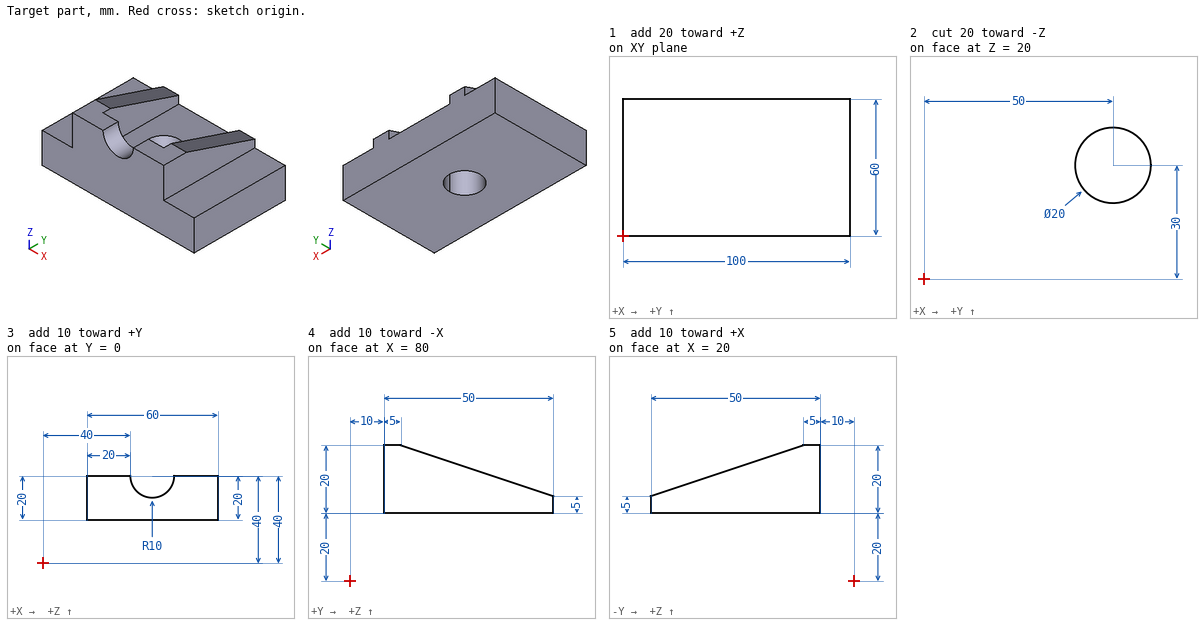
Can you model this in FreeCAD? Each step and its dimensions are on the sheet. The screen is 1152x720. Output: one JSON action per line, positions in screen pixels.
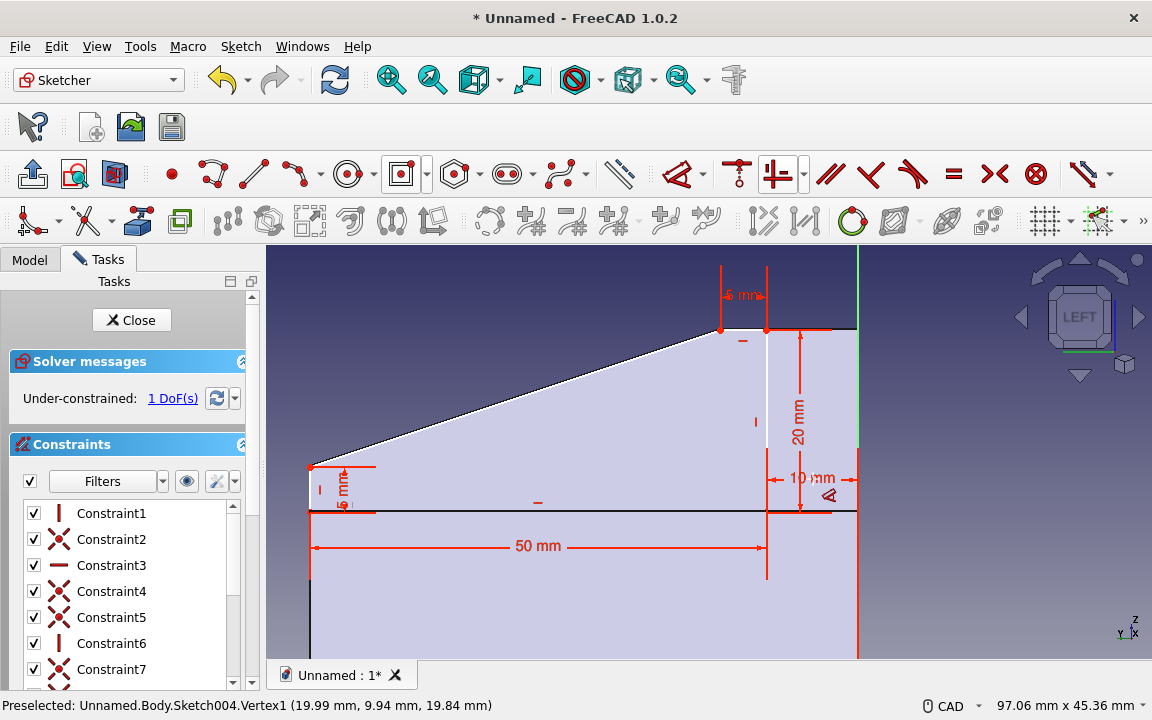
{"action": "left_click", "coordinate": [767, 513]}
{"action": "left_click", "coordinate": [892, 572]}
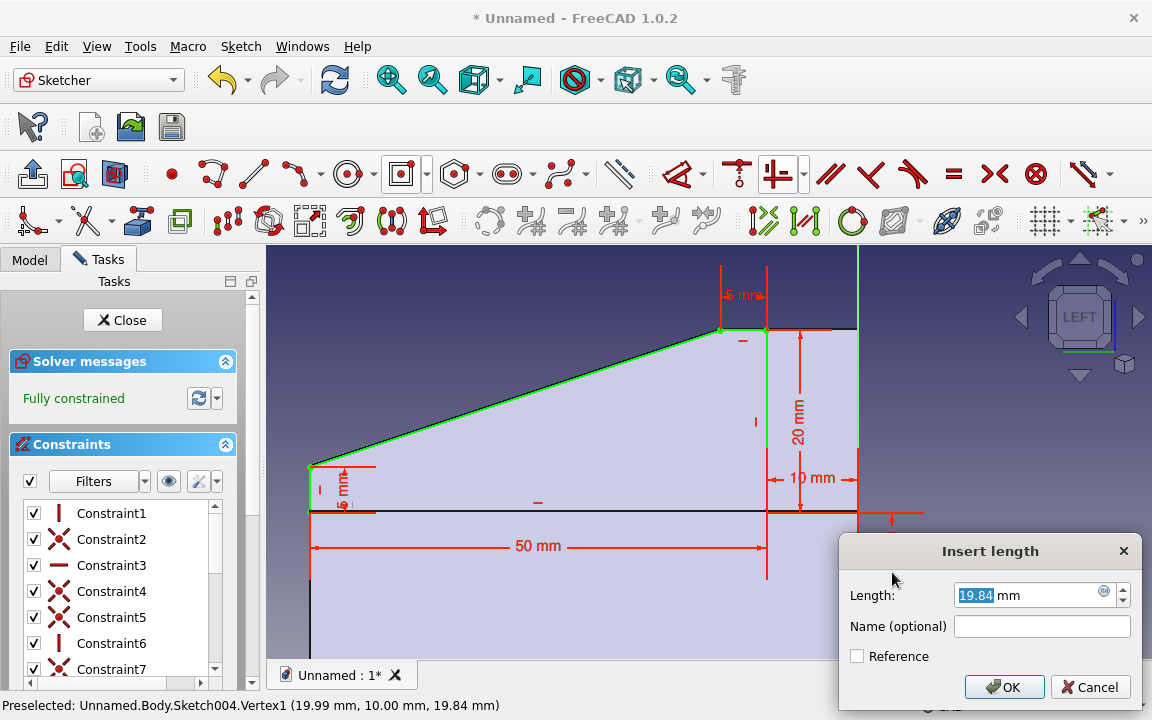
{"action": "type", "text": "20"}
{"action": "key", "text": "Return"}
{"action": "key", "text": "Escape"}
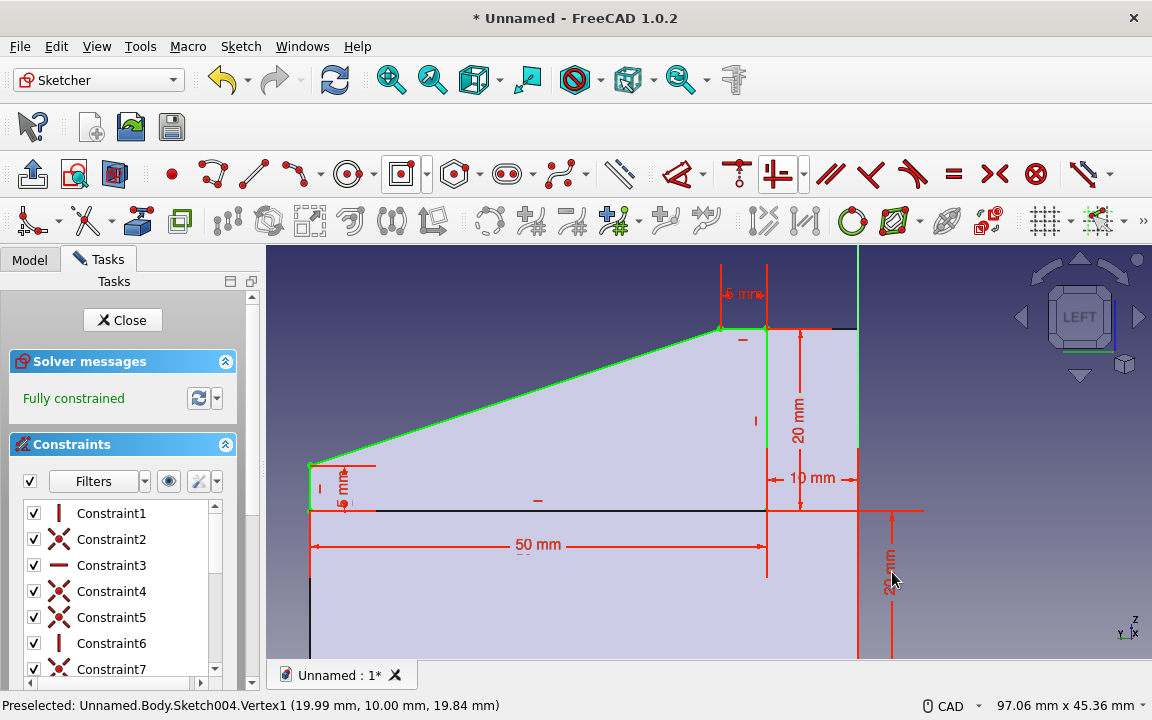
{"action": "left_click", "coordinate": [123, 320]}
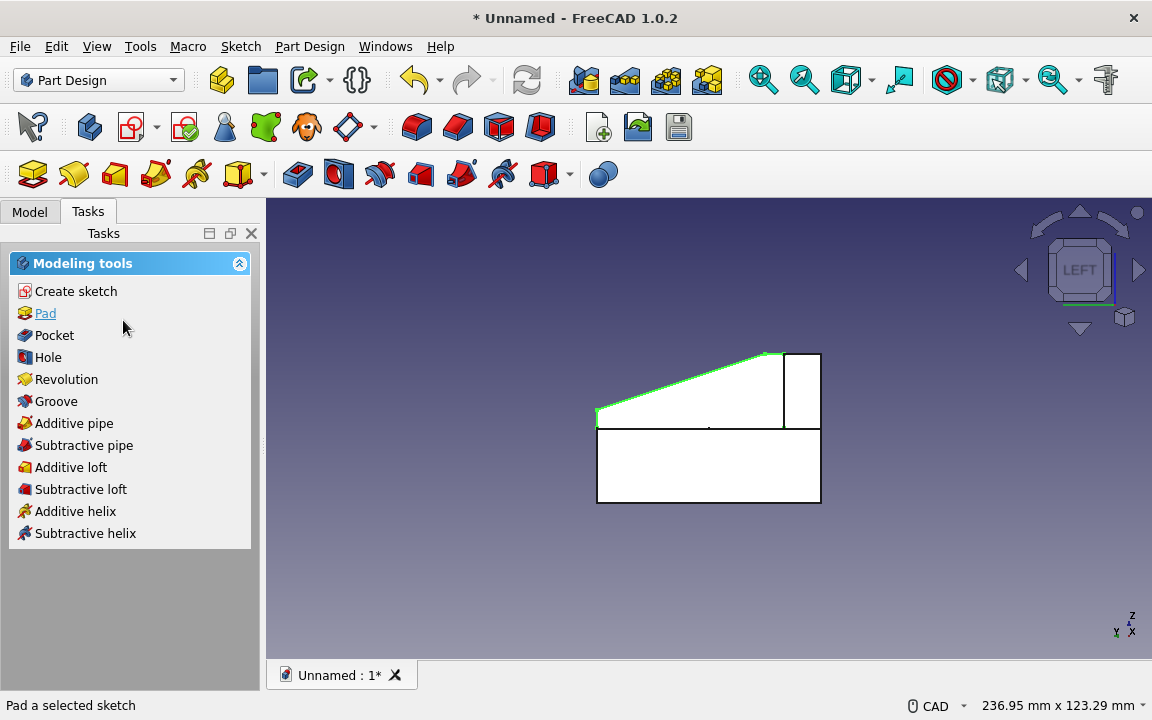
{"action": "left_click", "coordinate": [33, 174]}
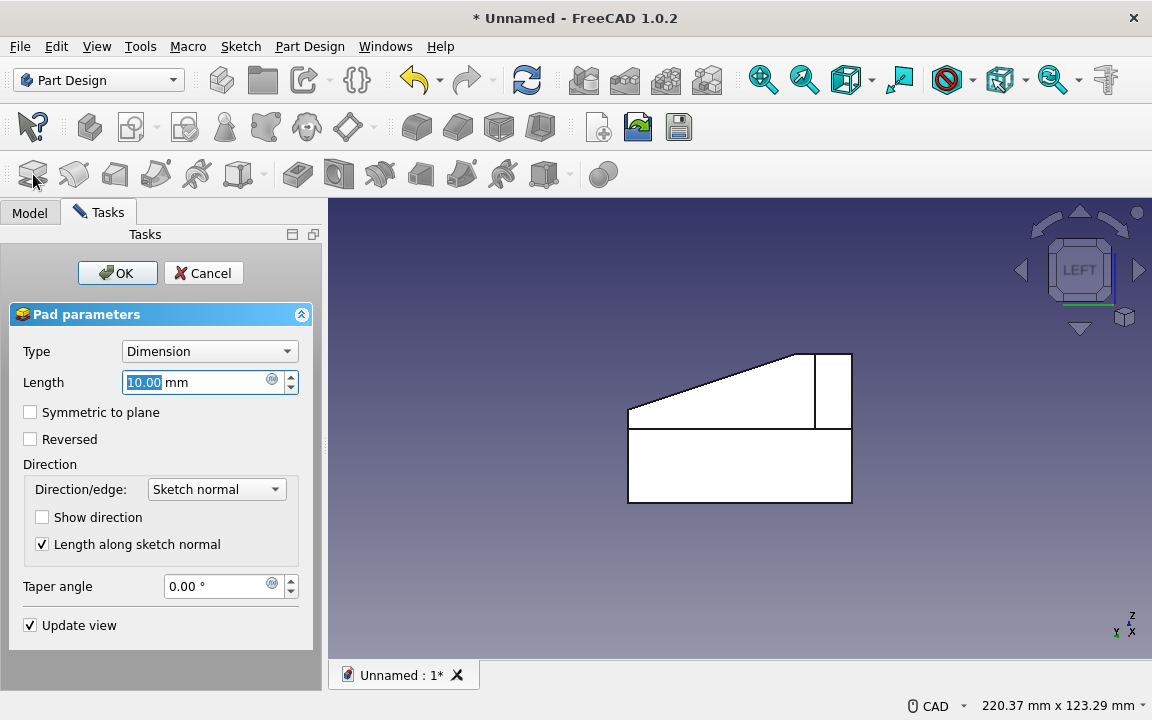
{"action": "type", "text": "10"}
{"action": "key", "text": "Tab"}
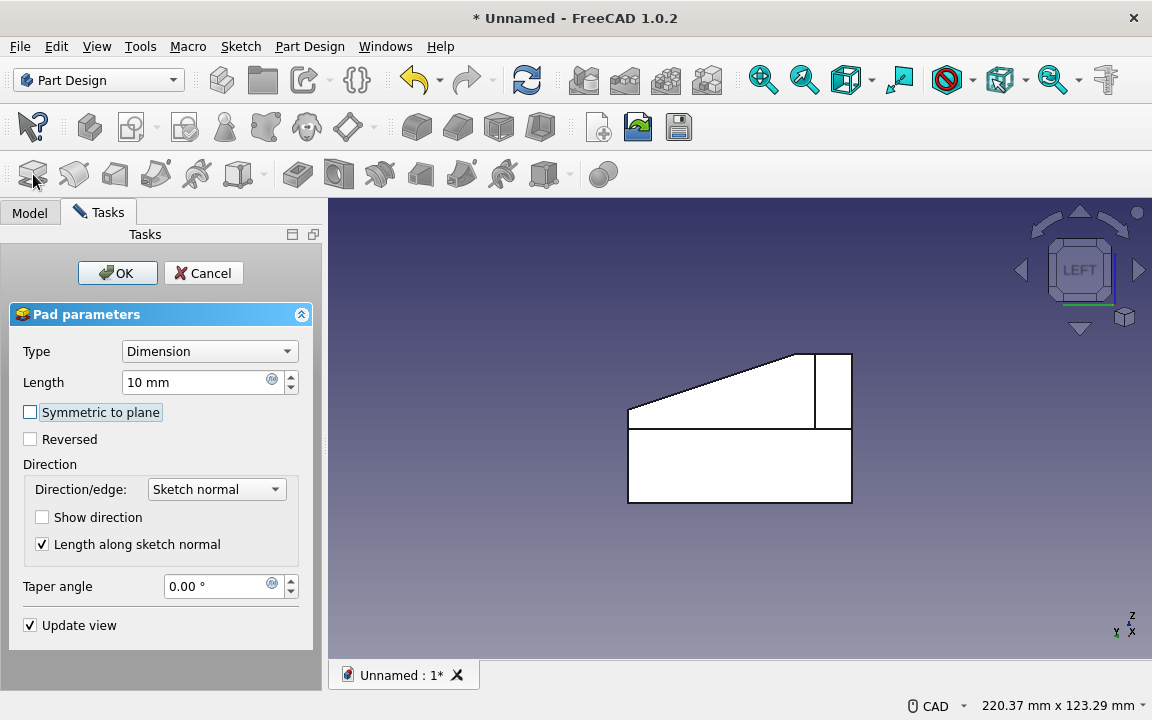
{"action": "left_click", "coordinate": [31, 439]}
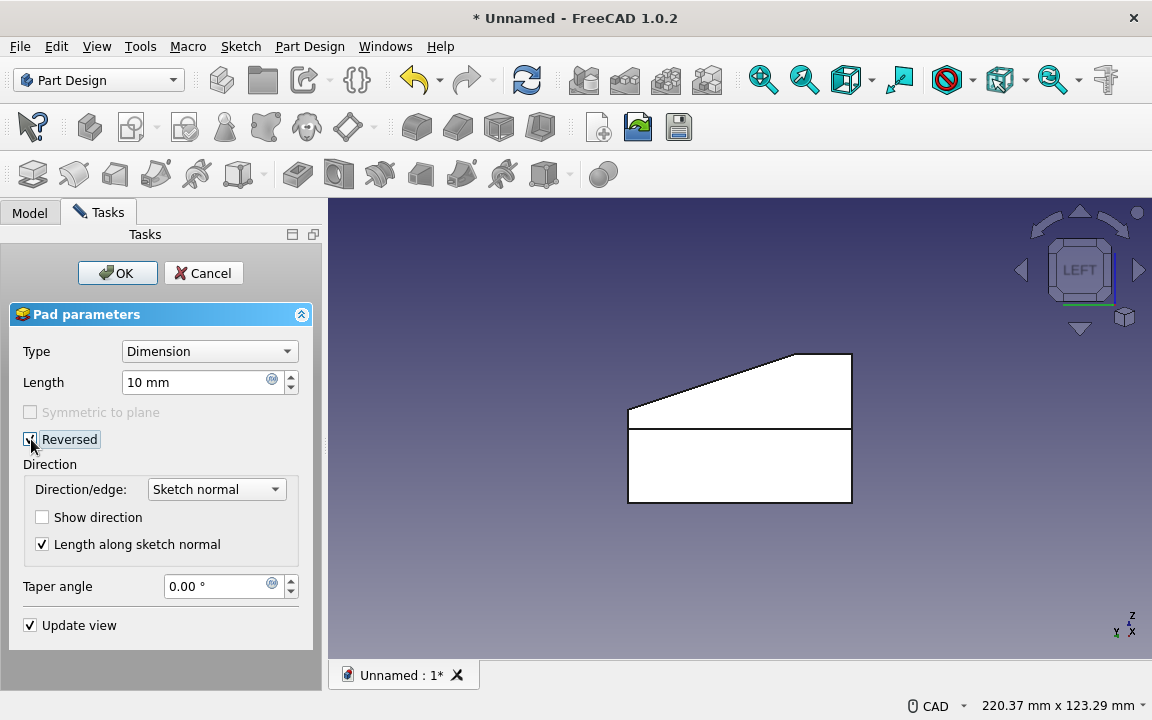
{"action": "left_click", "coordinate": [118, 273]}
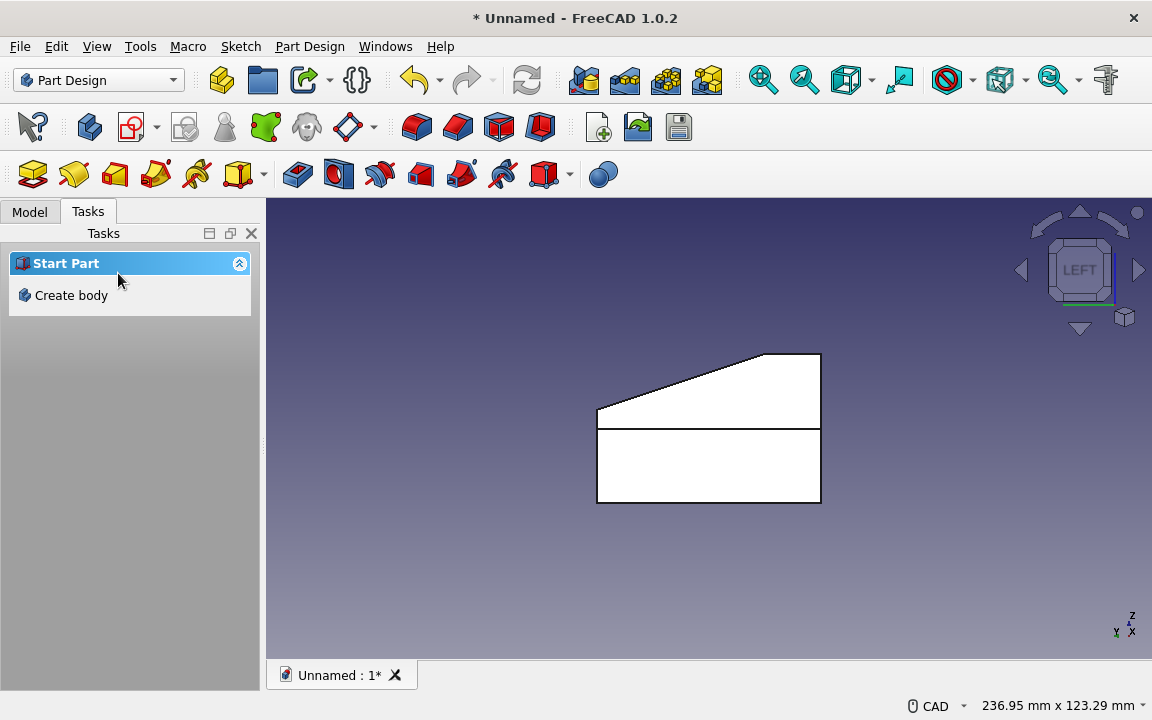
{"action": "key", "text": "0"}